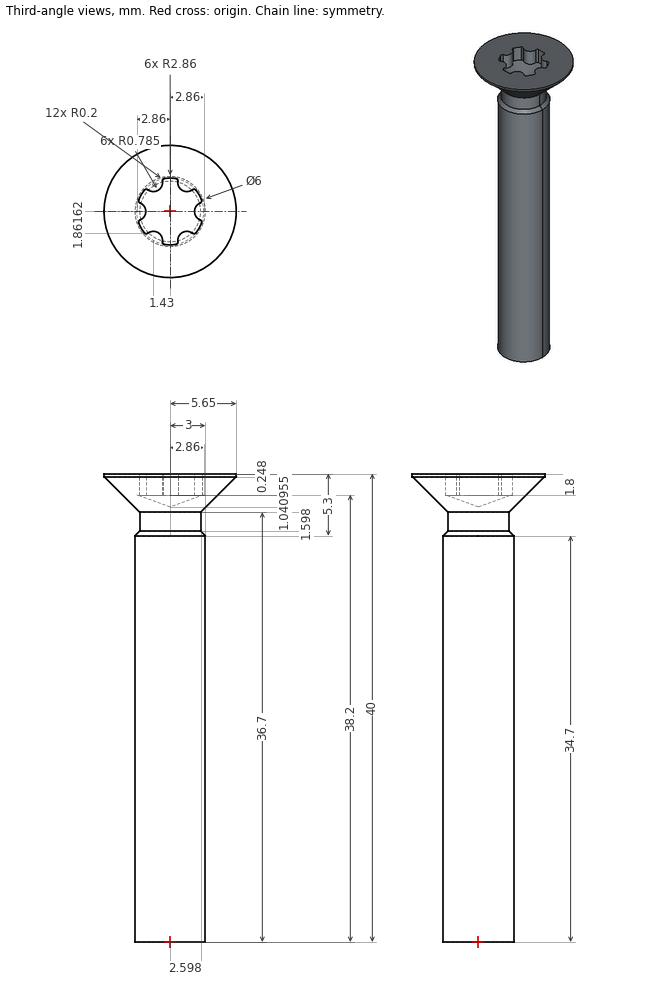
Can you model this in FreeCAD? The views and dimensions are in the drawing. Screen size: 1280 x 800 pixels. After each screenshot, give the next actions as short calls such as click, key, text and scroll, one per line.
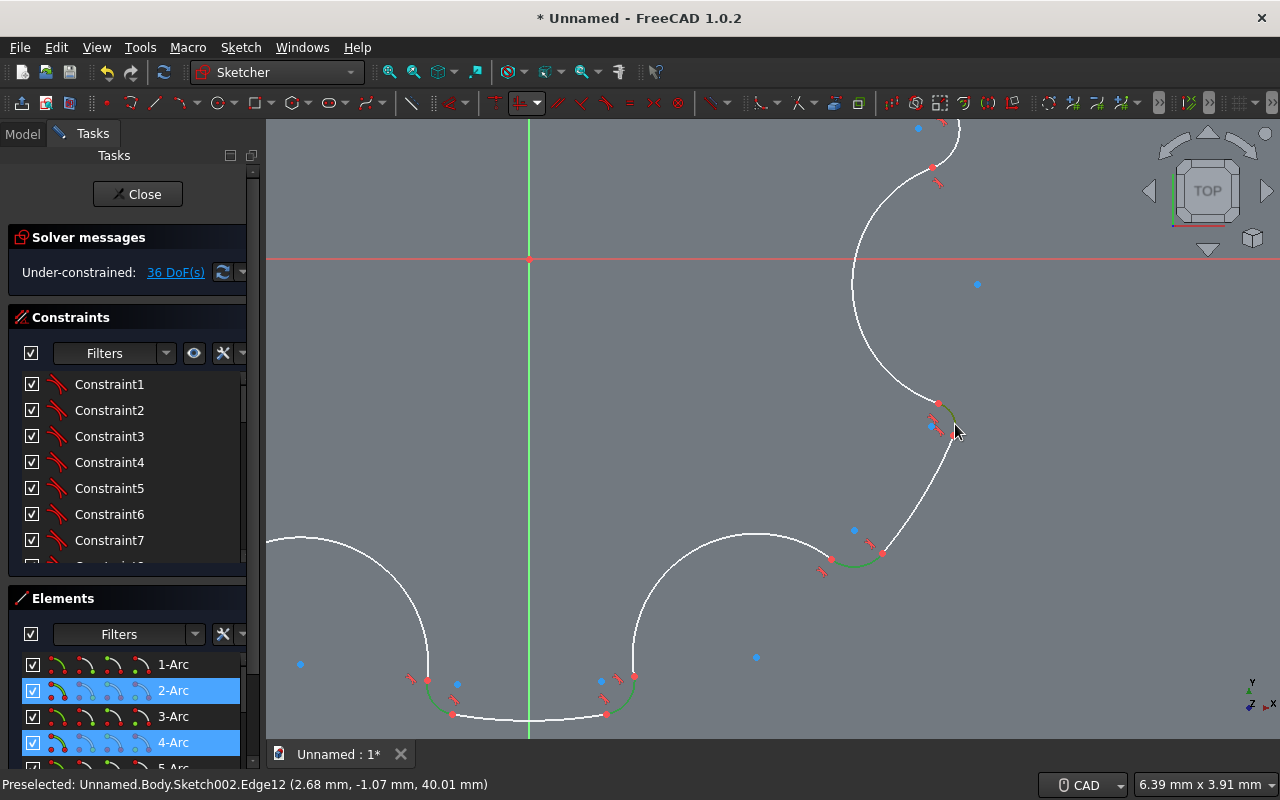
click(949, 157)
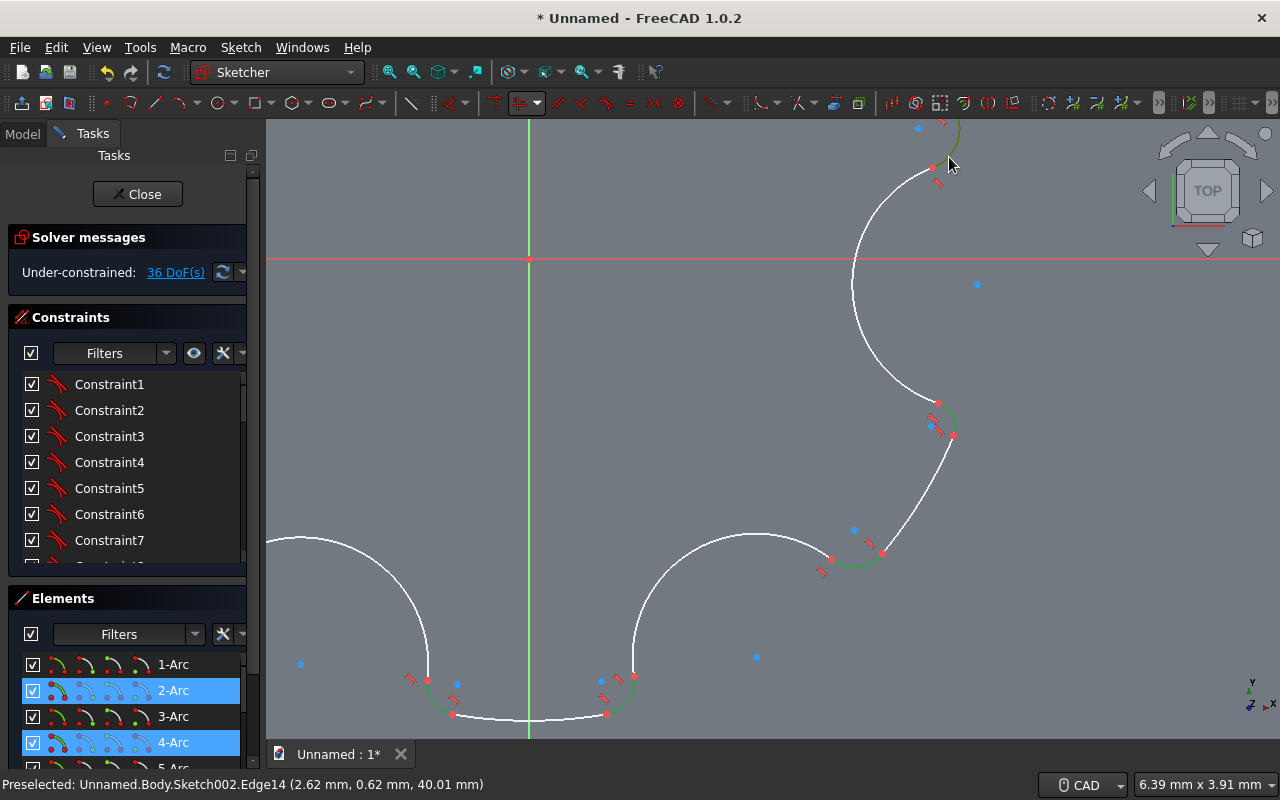
scroll(847, 567, down, 4)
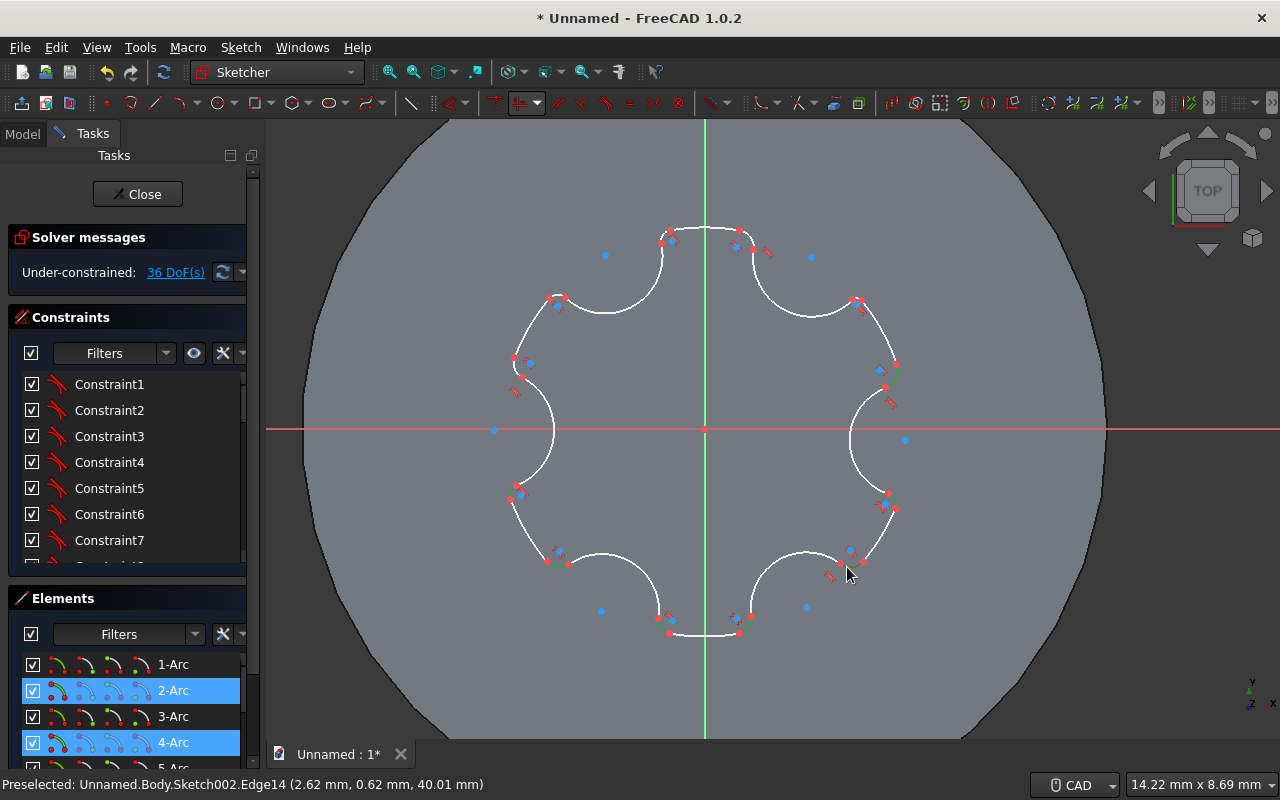
scroll(857, 298, up, 6)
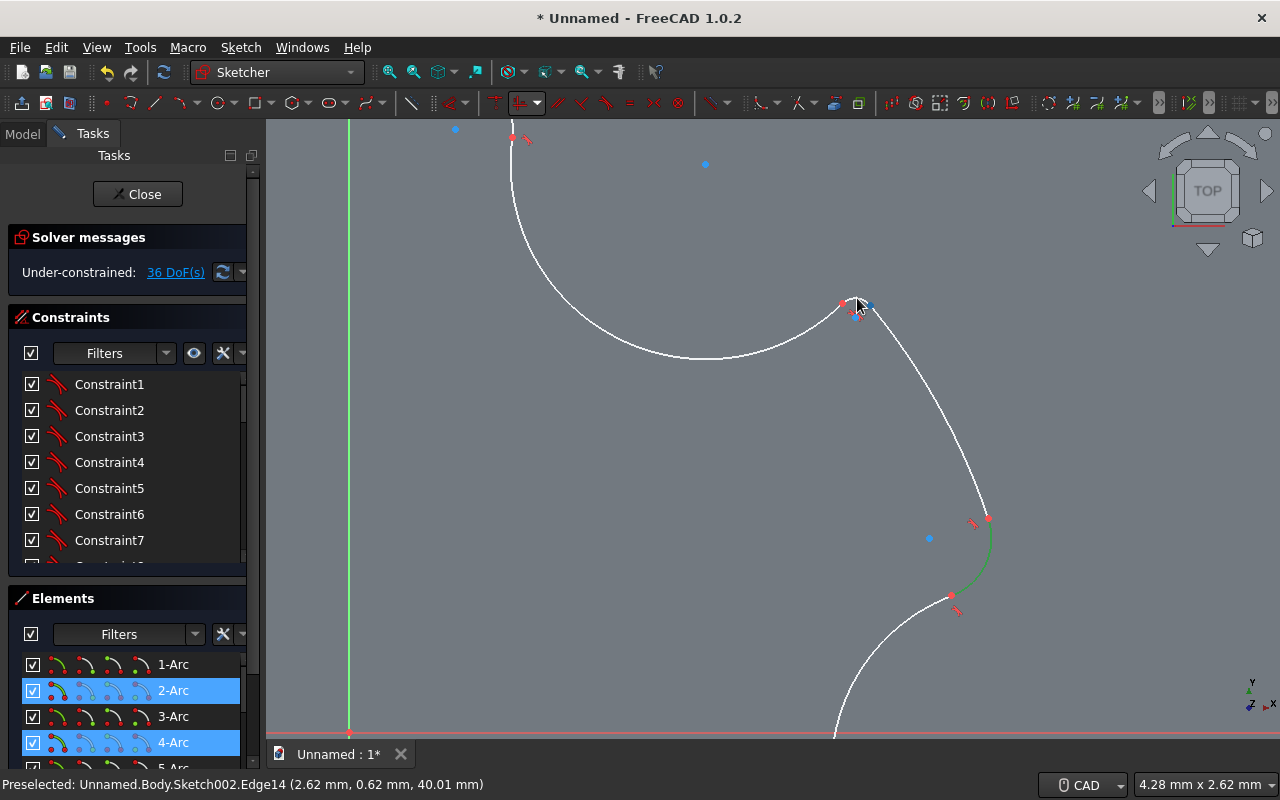
click(857, 298)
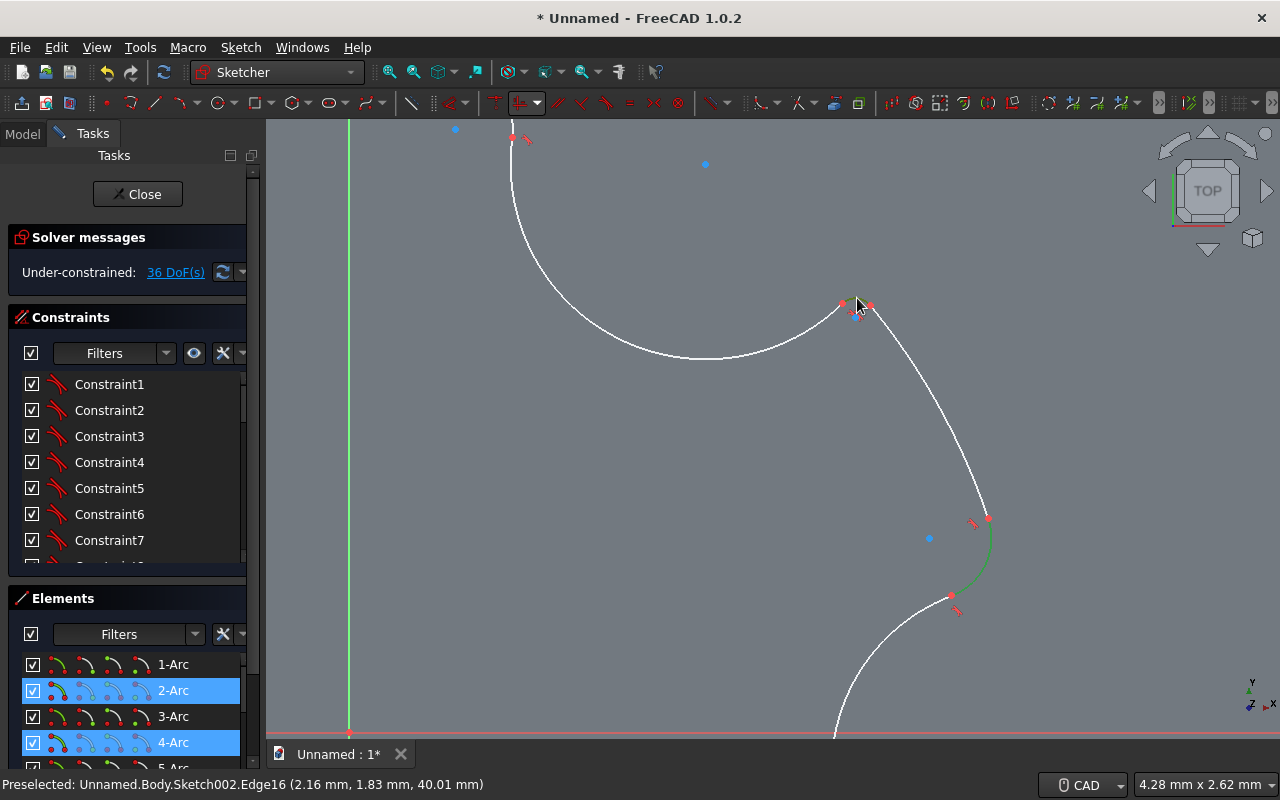
scroll(858, 298, down, 6)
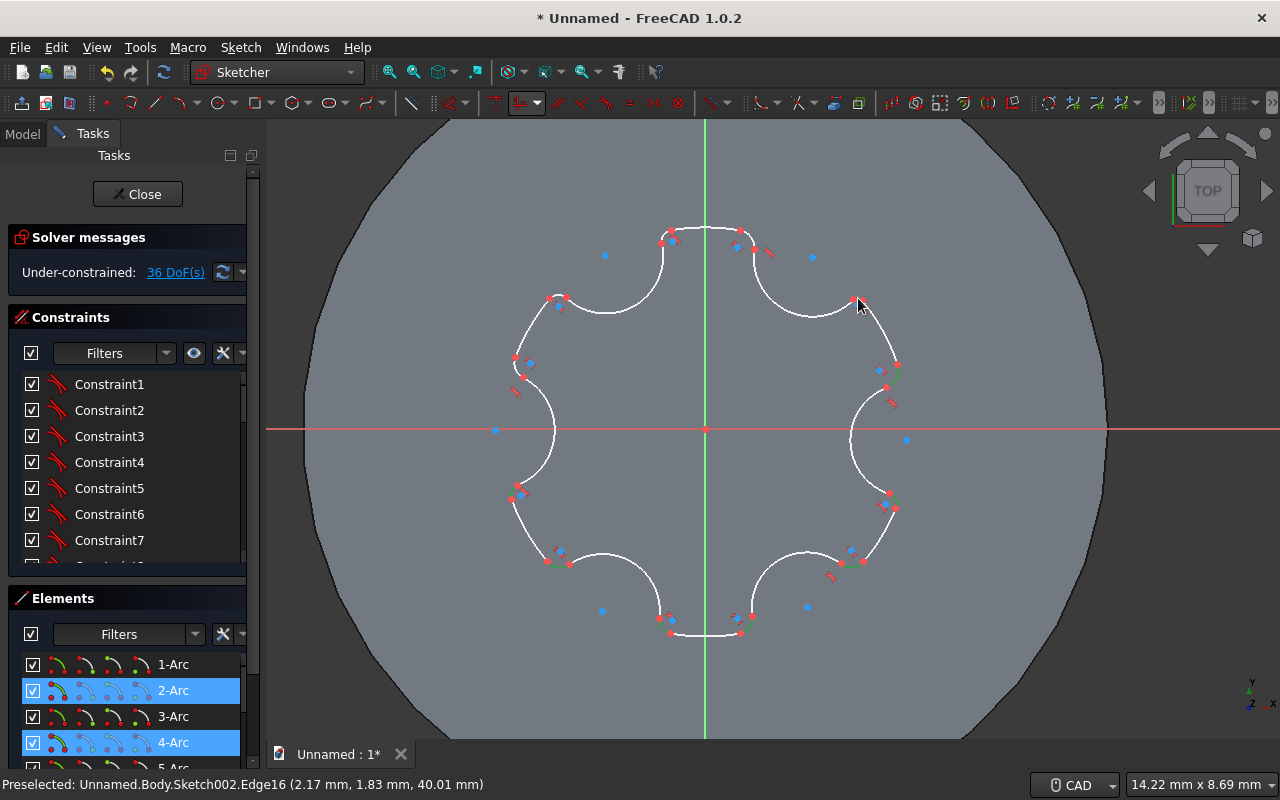
scroll(754, 242, up, 3)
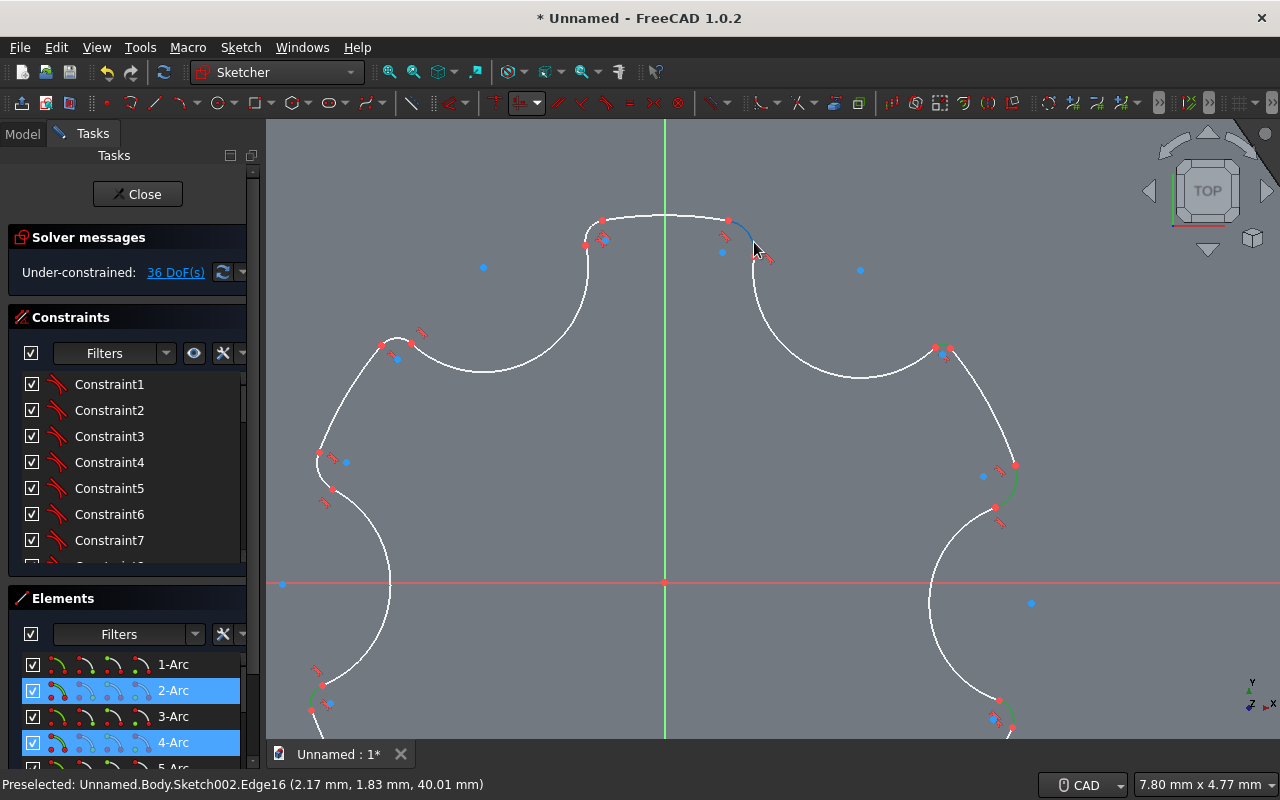
click(753, 242)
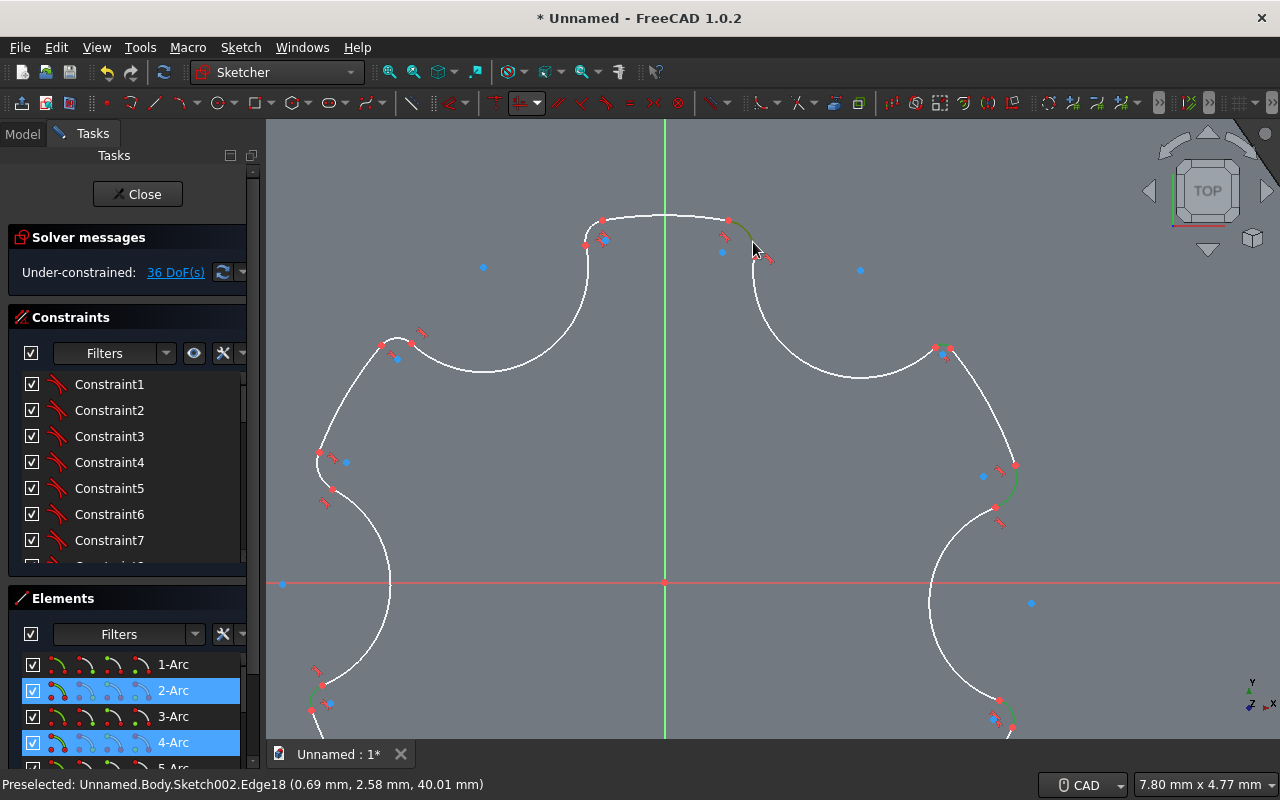
scroll(593, 225, up, 2)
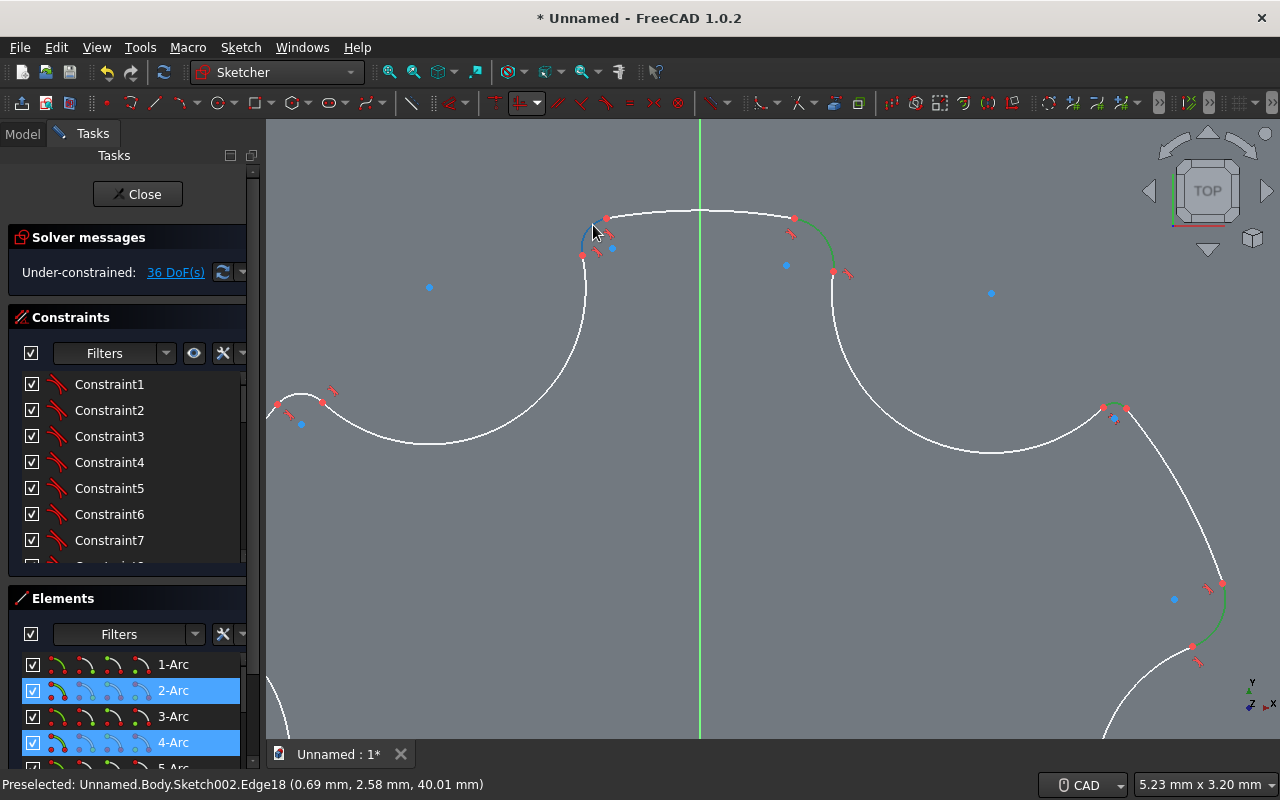
click(594, 224)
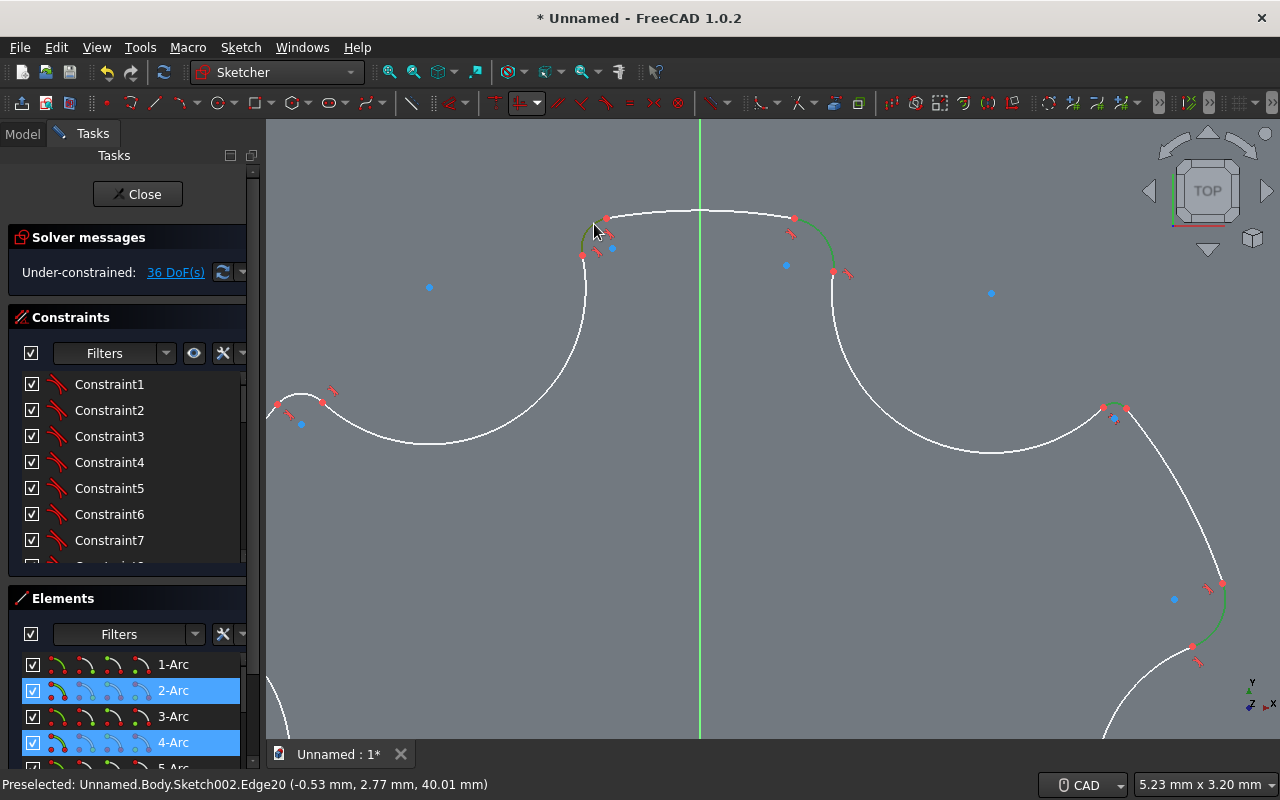
click(309, 395)